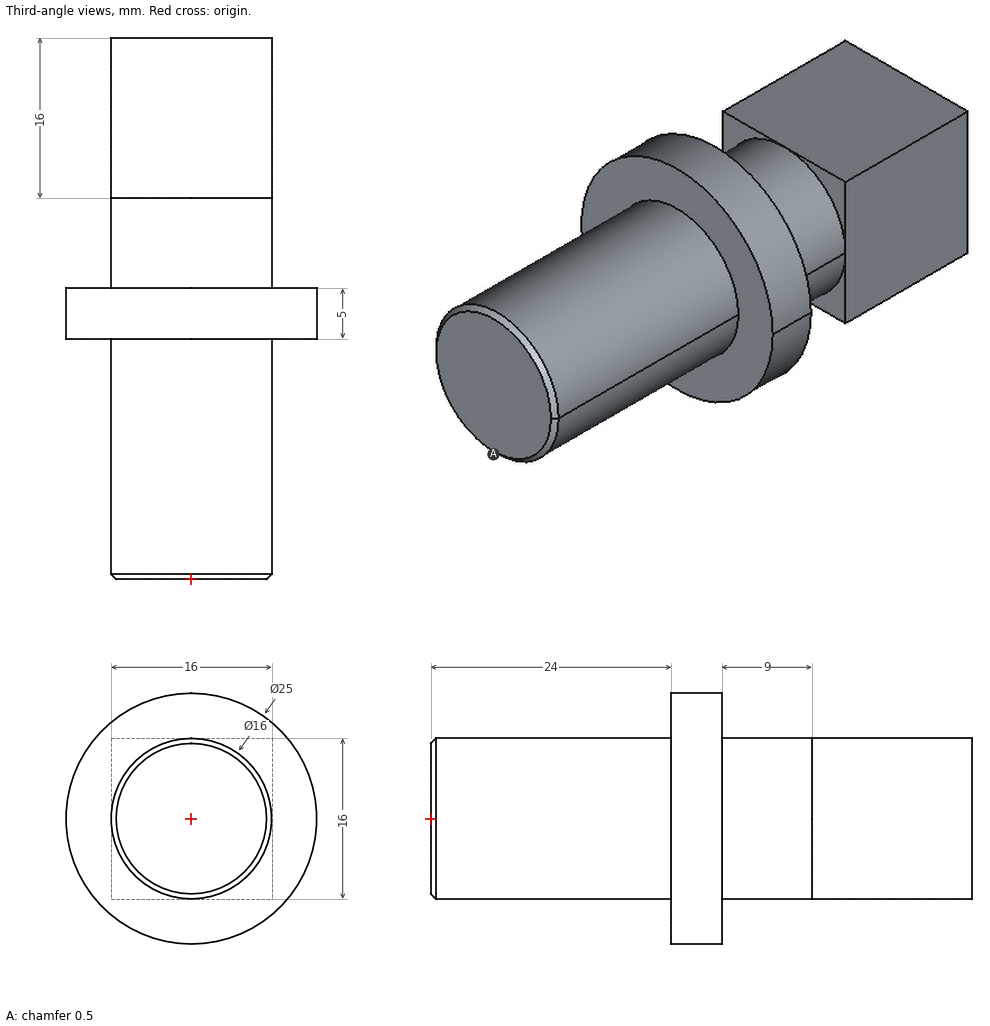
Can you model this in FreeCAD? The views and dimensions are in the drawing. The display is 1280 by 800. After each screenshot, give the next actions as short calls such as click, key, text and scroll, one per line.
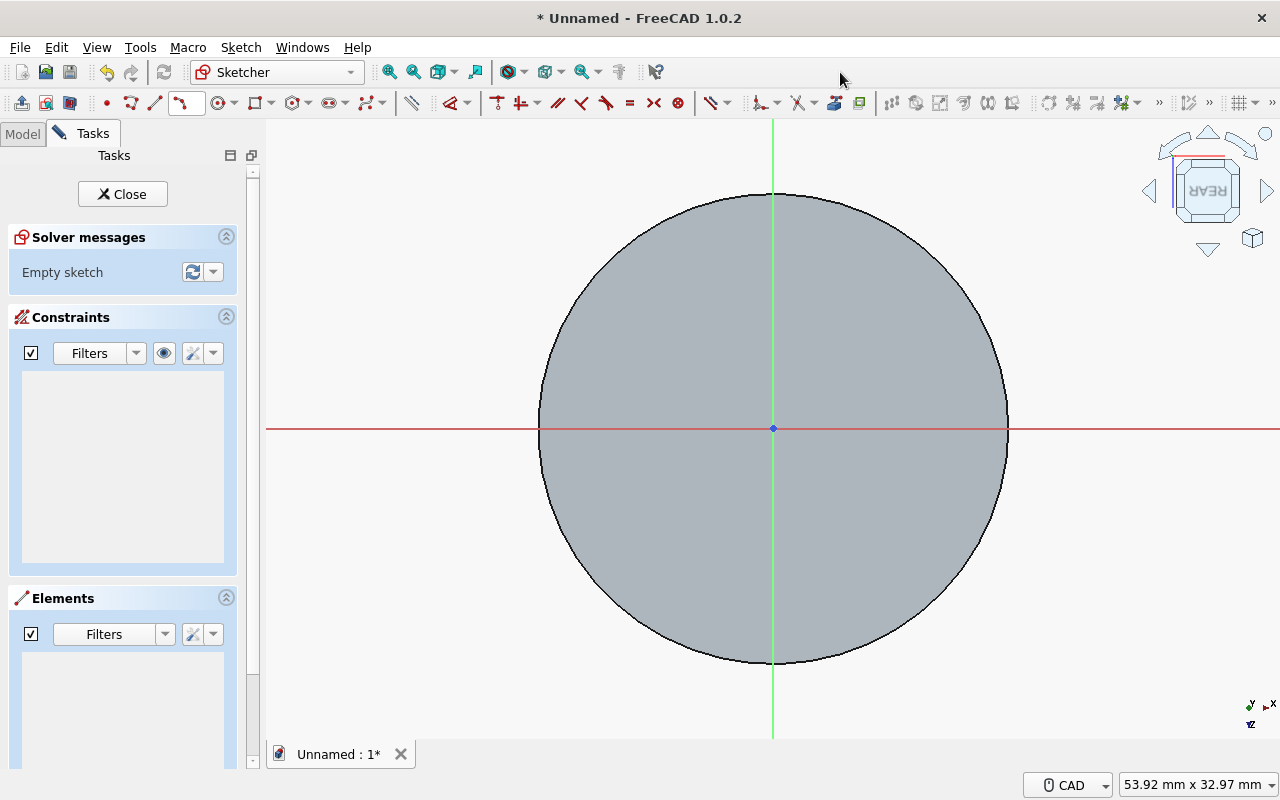
click(218, 104)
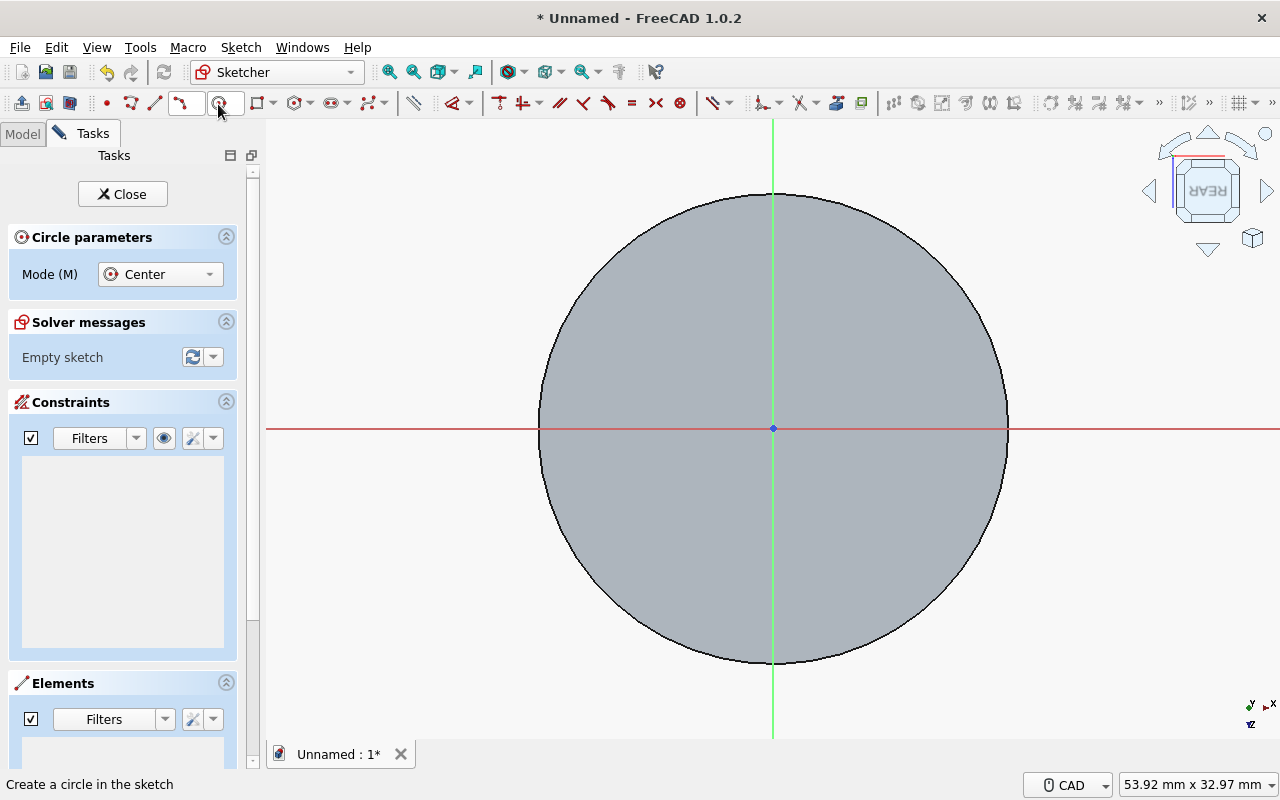
click(773, 429)
move(880, 323)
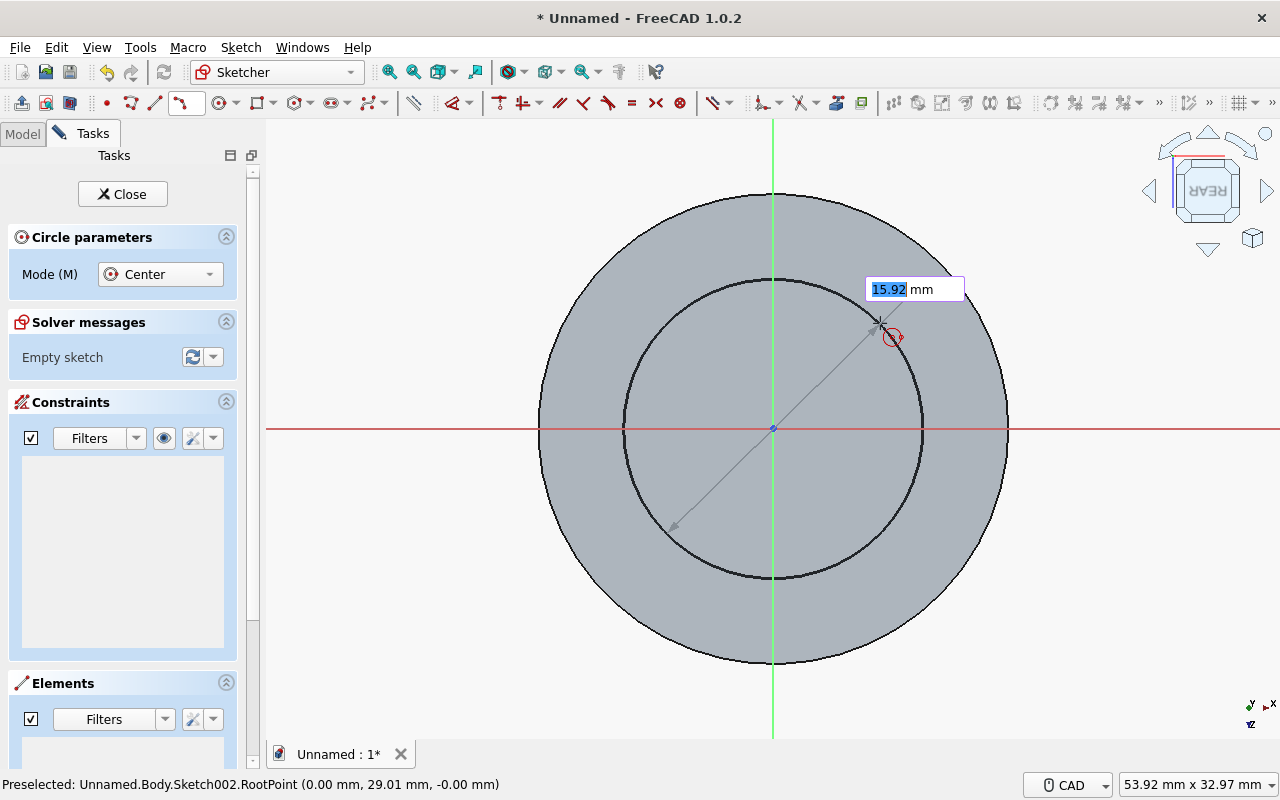
text(16)
key(Return)
key(Escape)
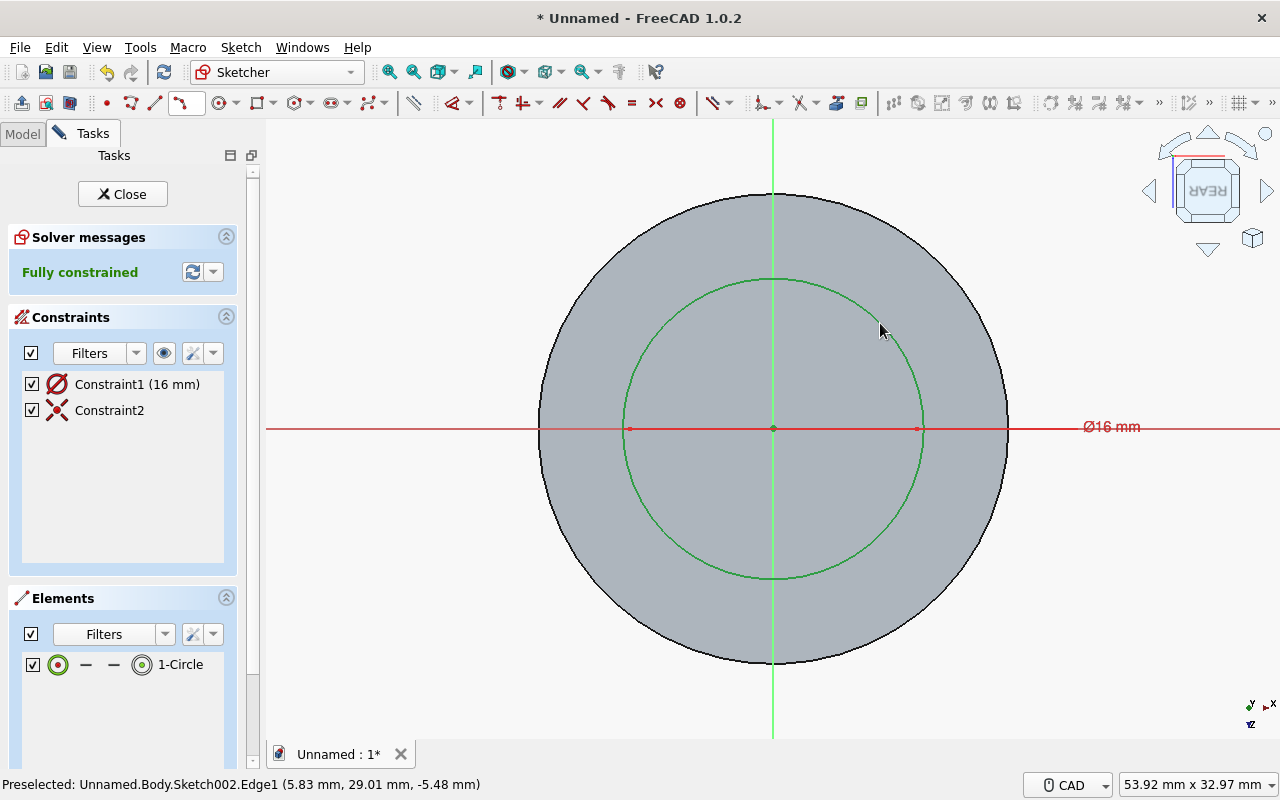
click(123, 194)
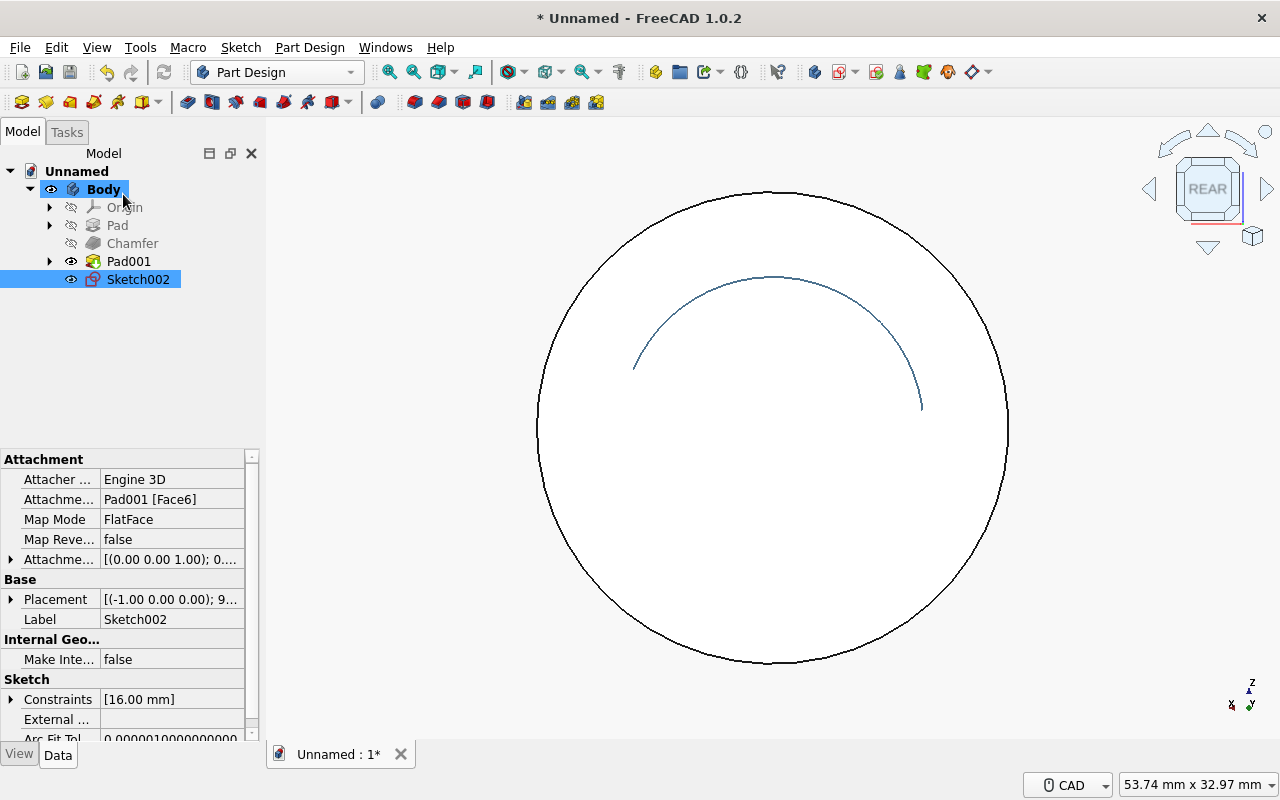
click(22, 102)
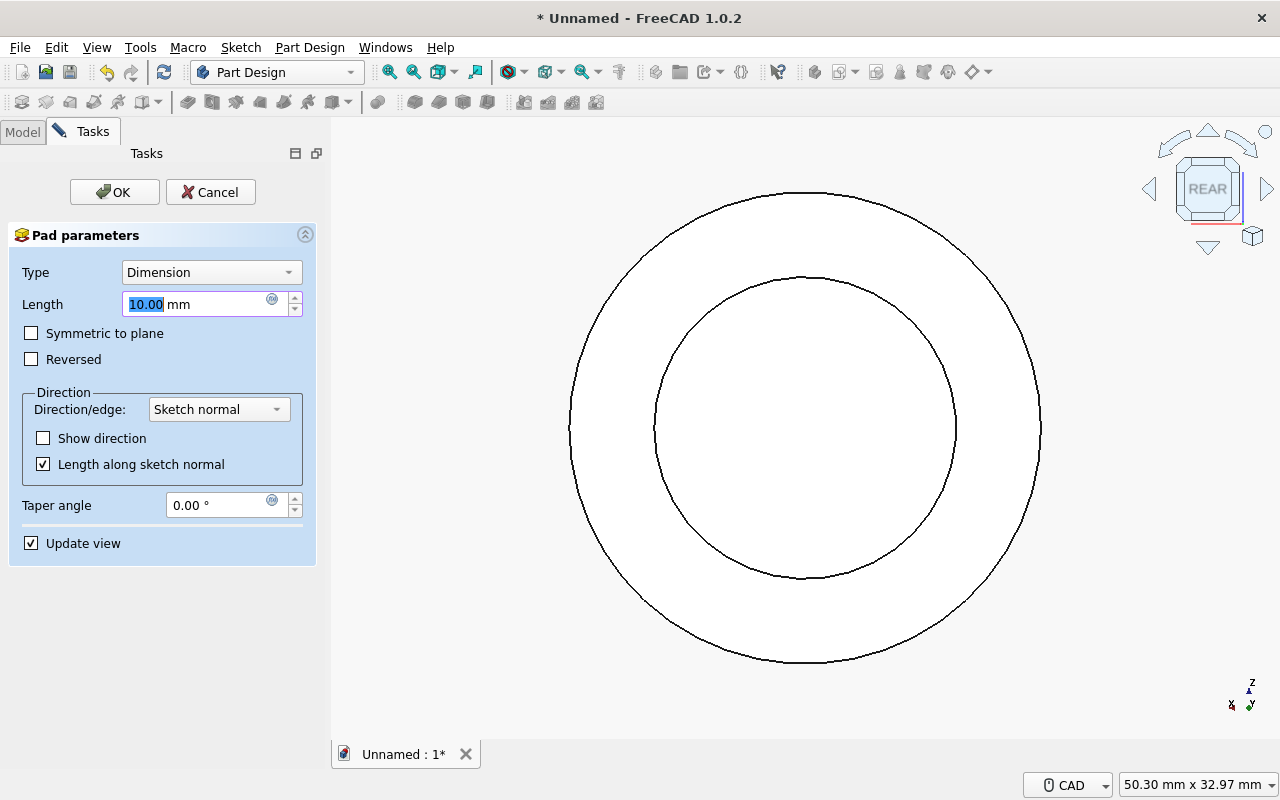
text(9)
key(Tab)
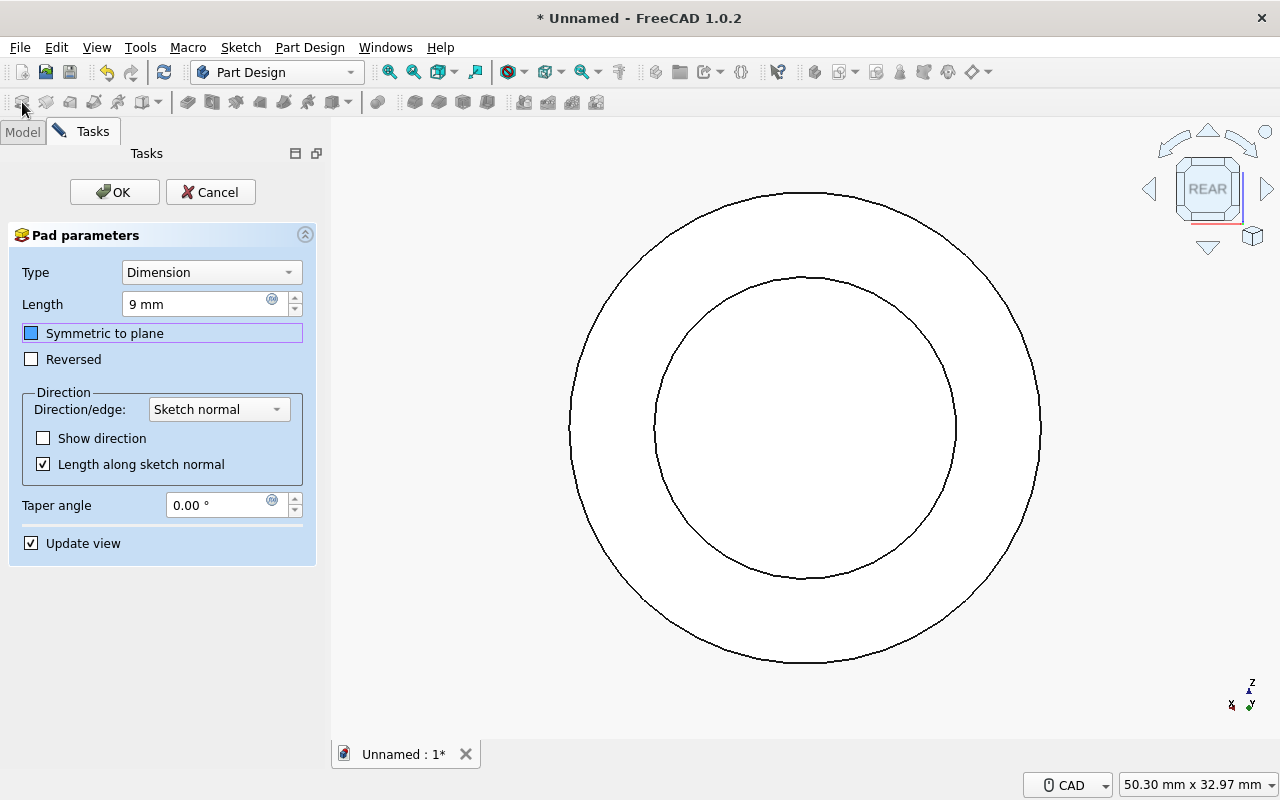
click(115, 192)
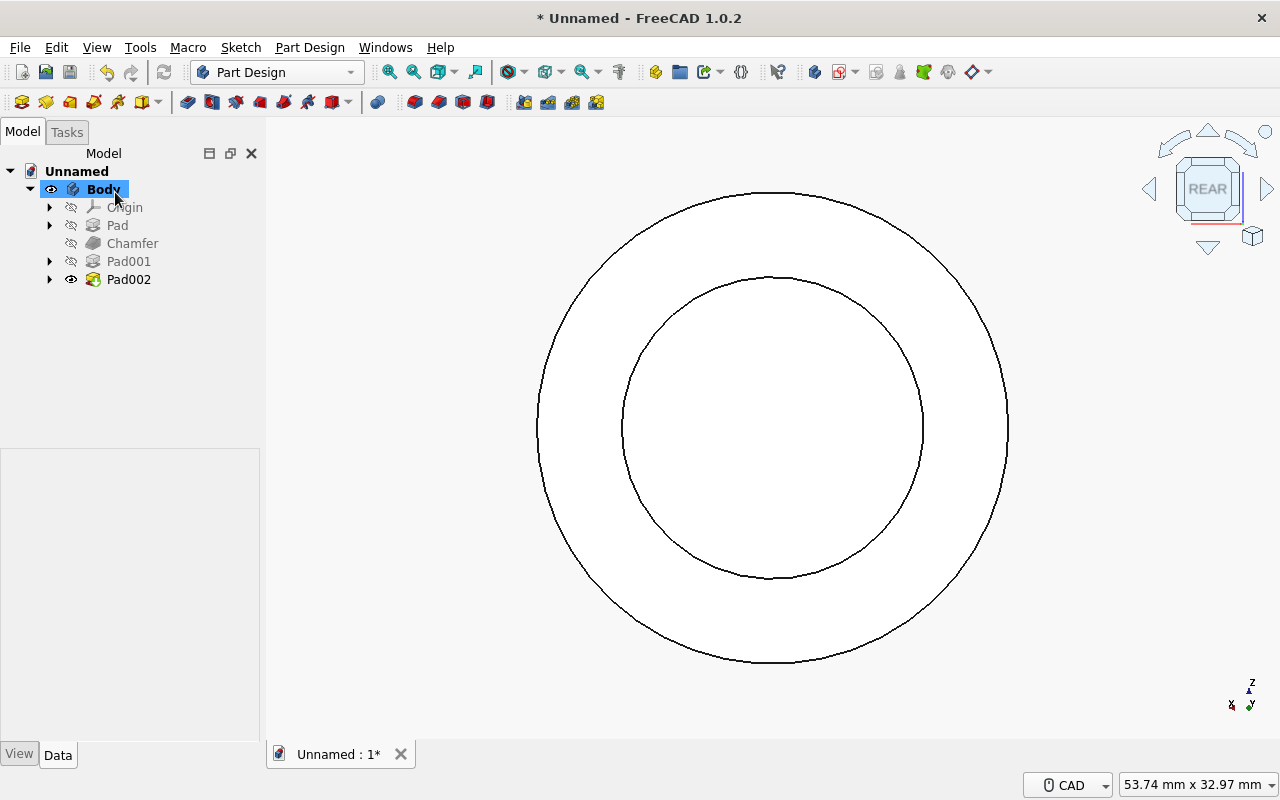
click(773, 427)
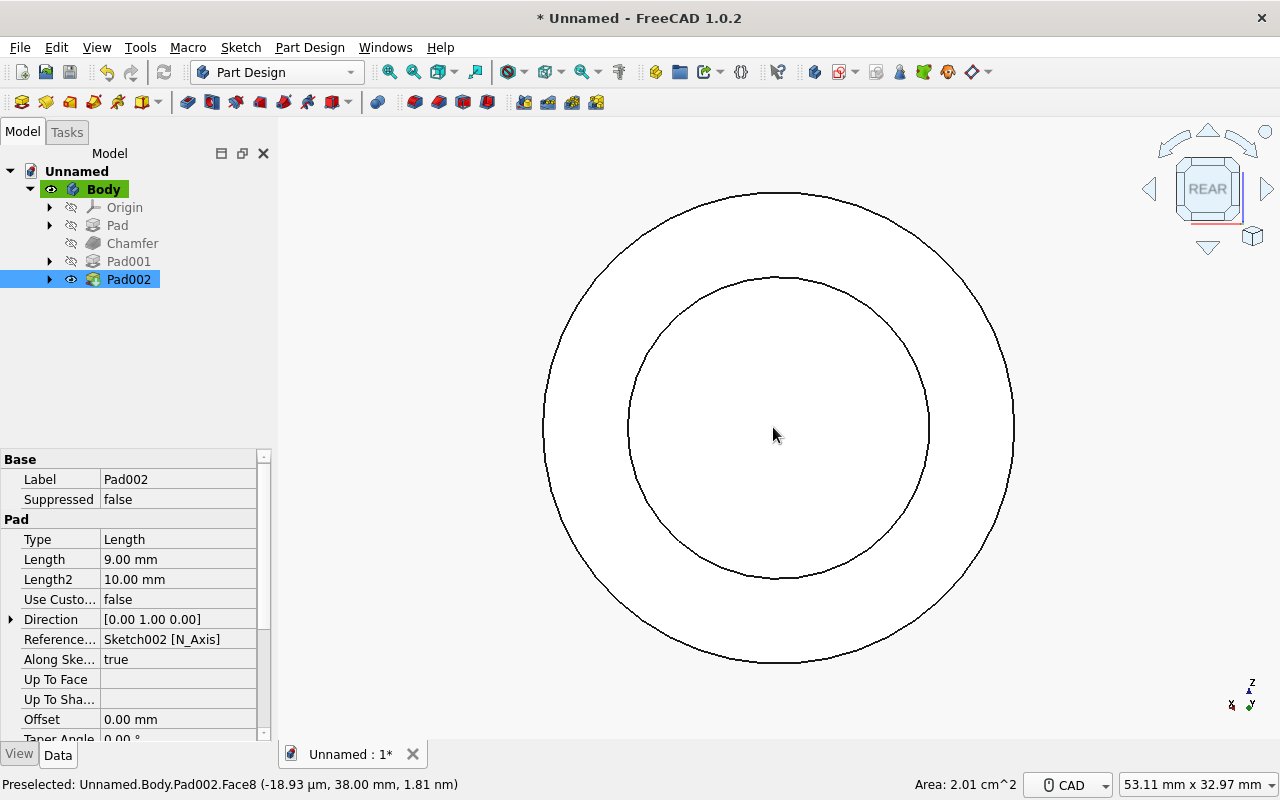
click(840, 72)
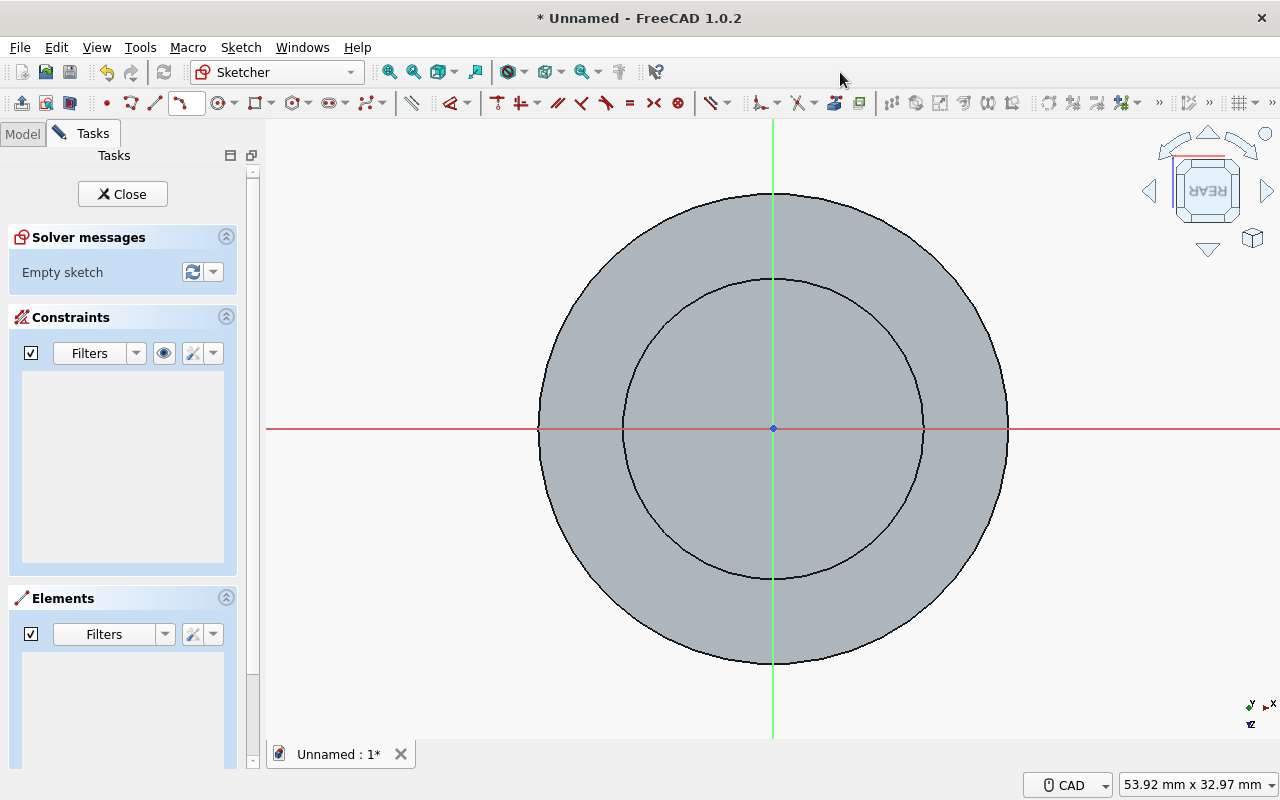
click(274, 104)